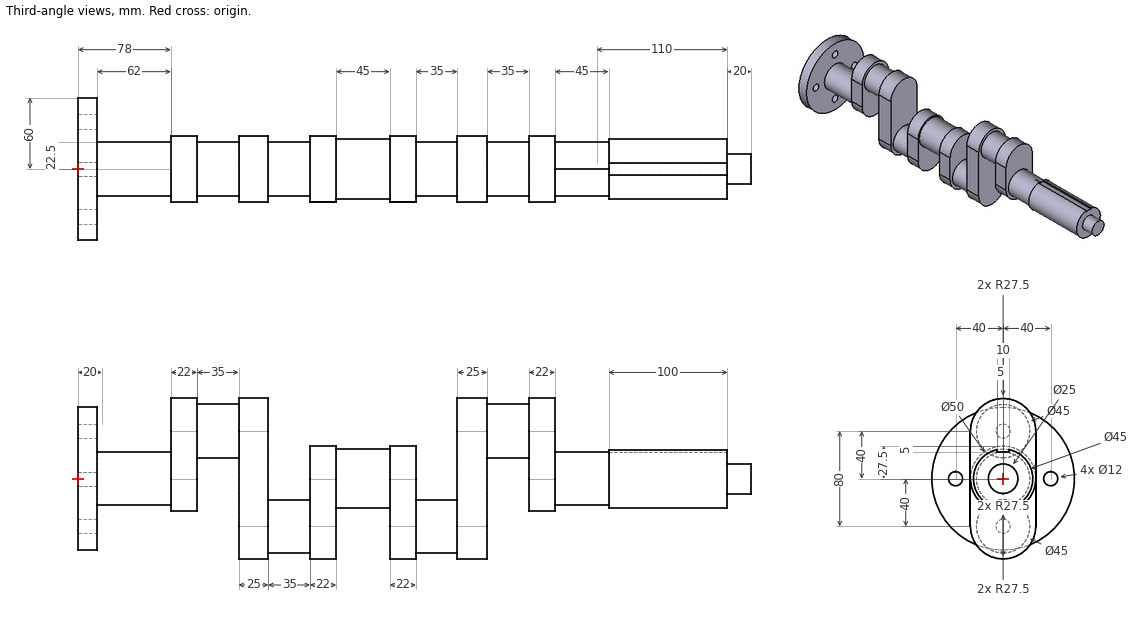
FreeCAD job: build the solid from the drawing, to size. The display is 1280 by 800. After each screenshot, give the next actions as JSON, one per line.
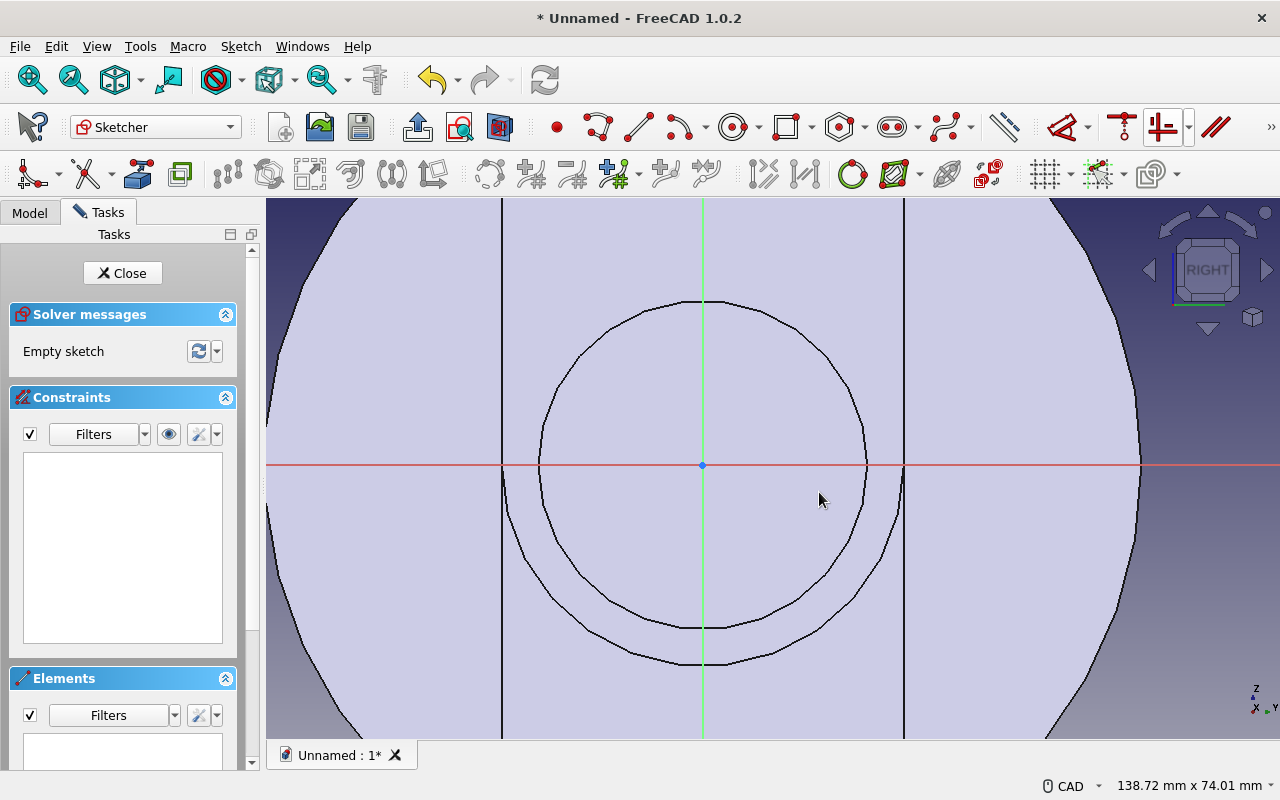
{"action": "left_click", "coordinate": [732, 128]}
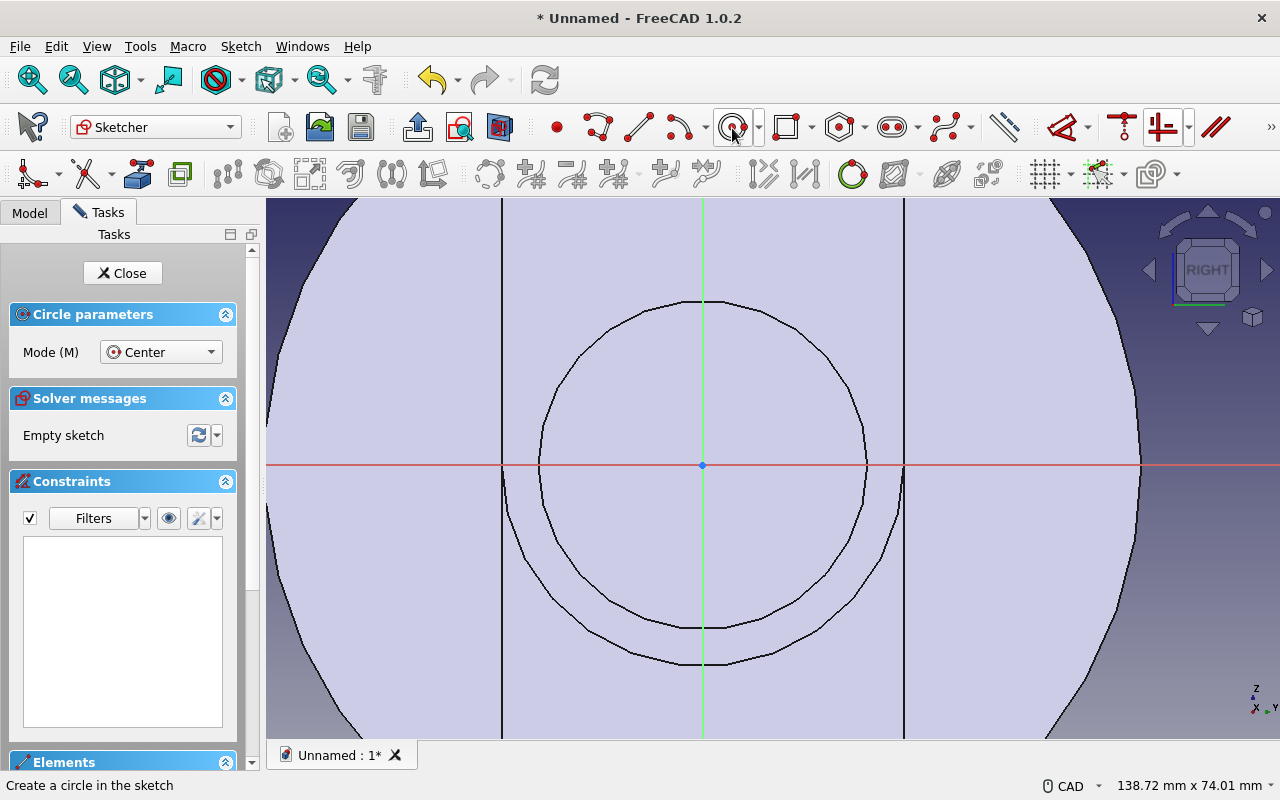
{"action": "left_click", "coordinate": [703, 465]}
{"action": "left_click", "coordinate": [832, 336]}
{"action": "key", "text": "Escape"}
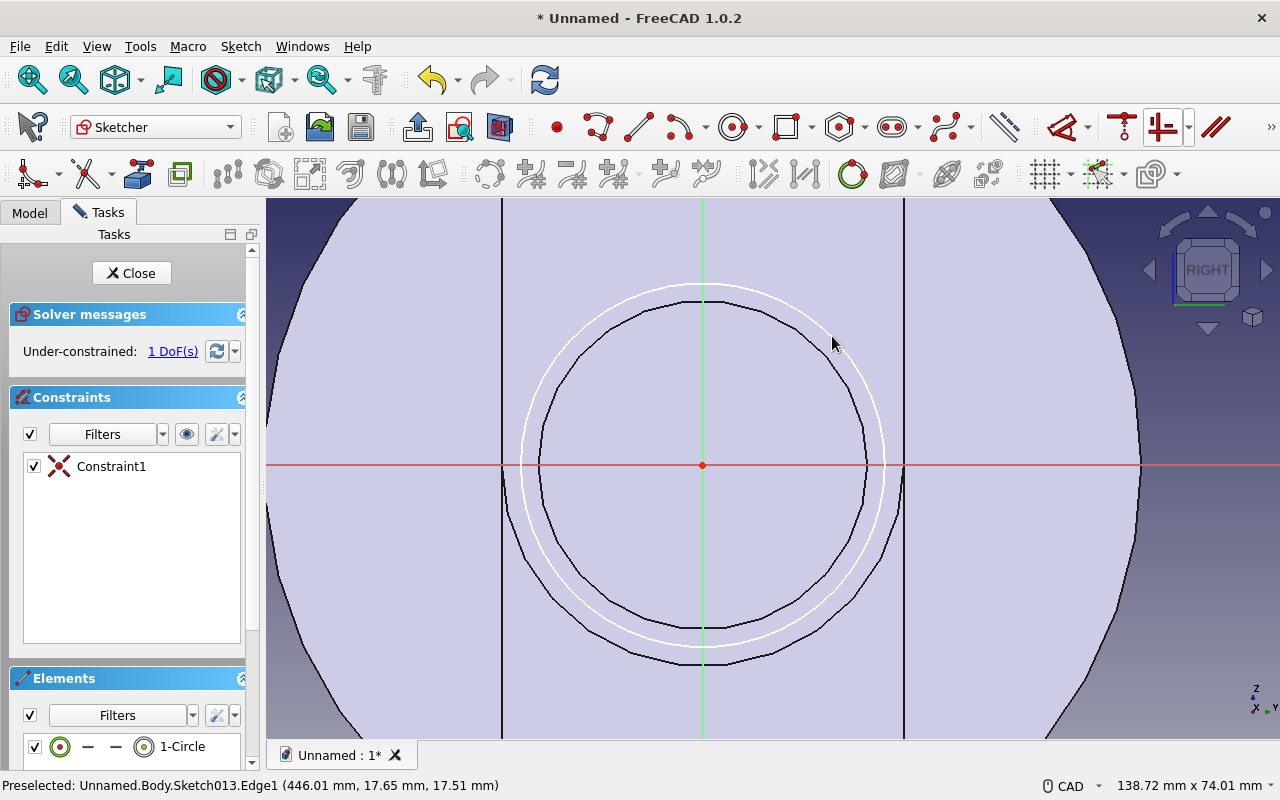
{"action": "key", "text": "d"}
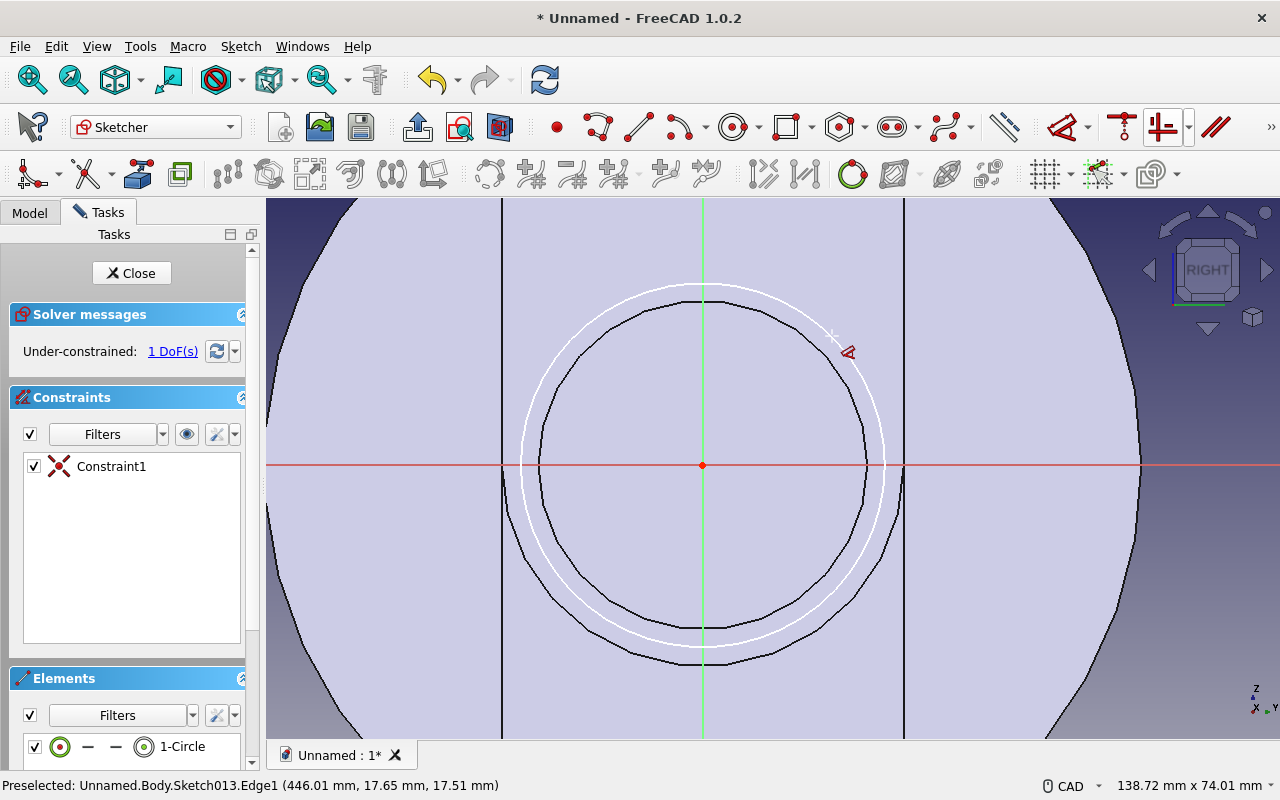
{"action": "left_click", "coordinate": [831, 336]}
{"action": "left_click", "coordinate": [854, 313]}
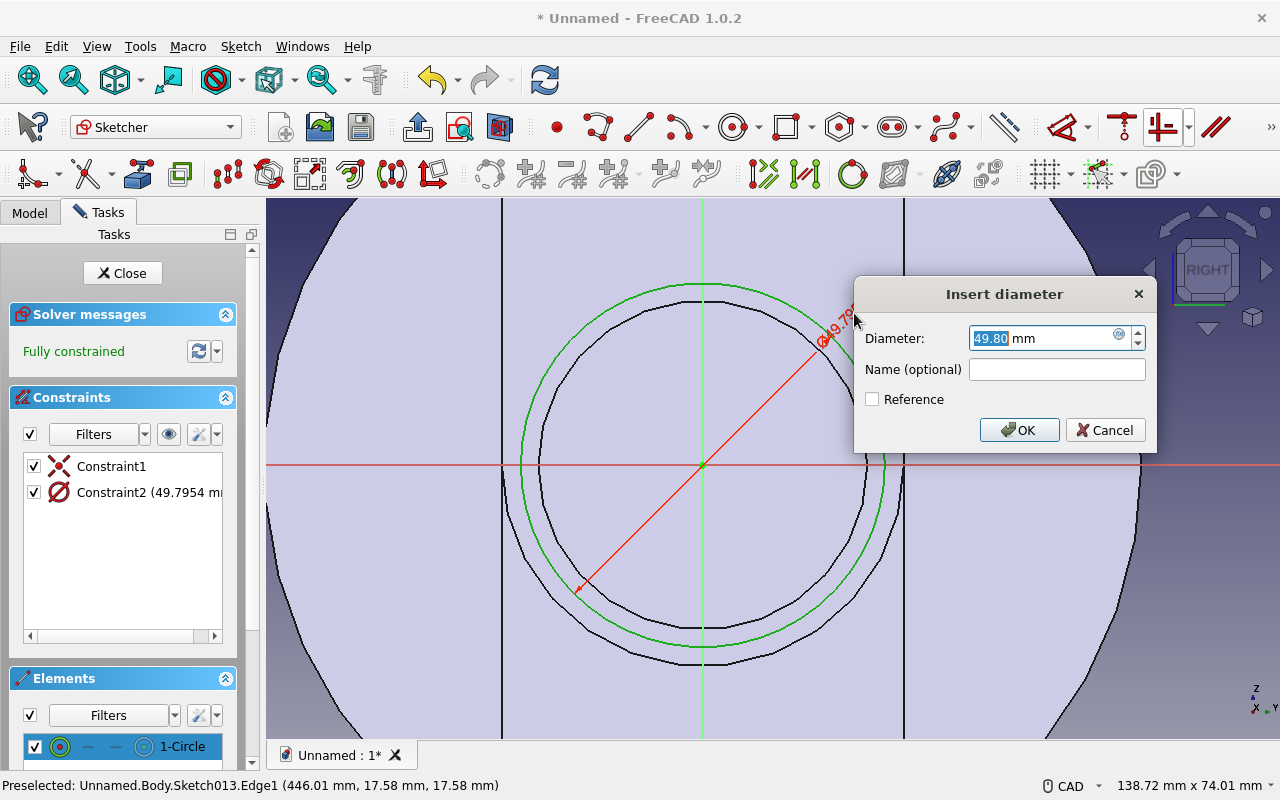
{"action": "type", "text": "50"}
{"action": "key", "text": "Return"}
{"action": "key", "text": "Escape"}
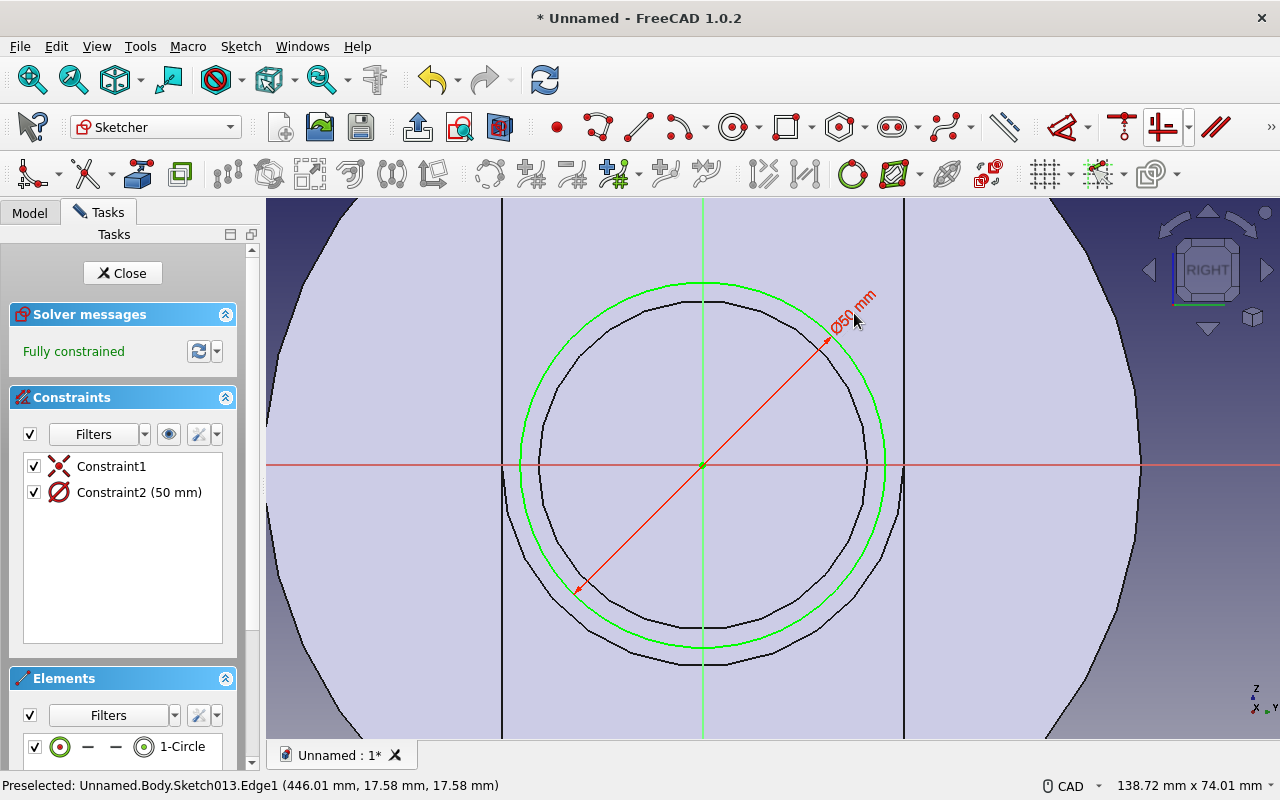
{"action": "left_click", "coordinate": [123, 273]}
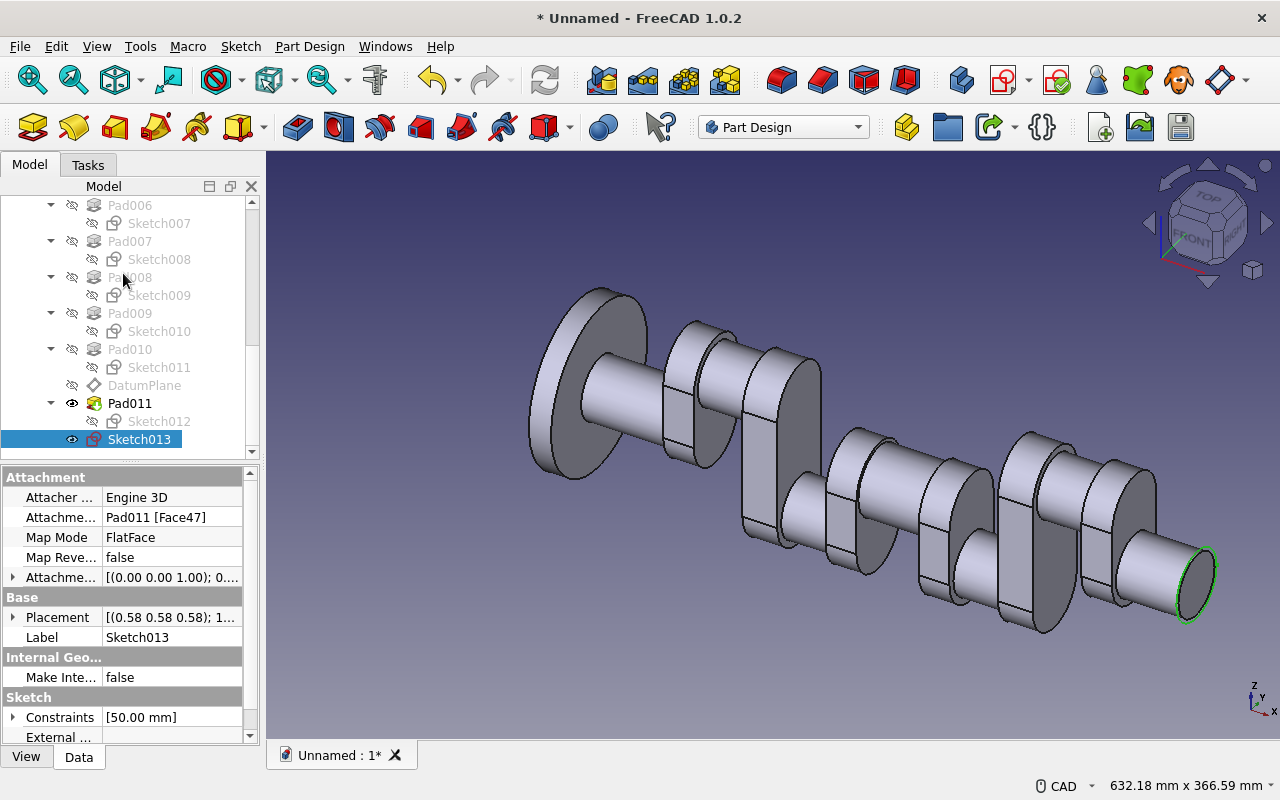
{"action": "left_click", "coordinate": [33, 128]}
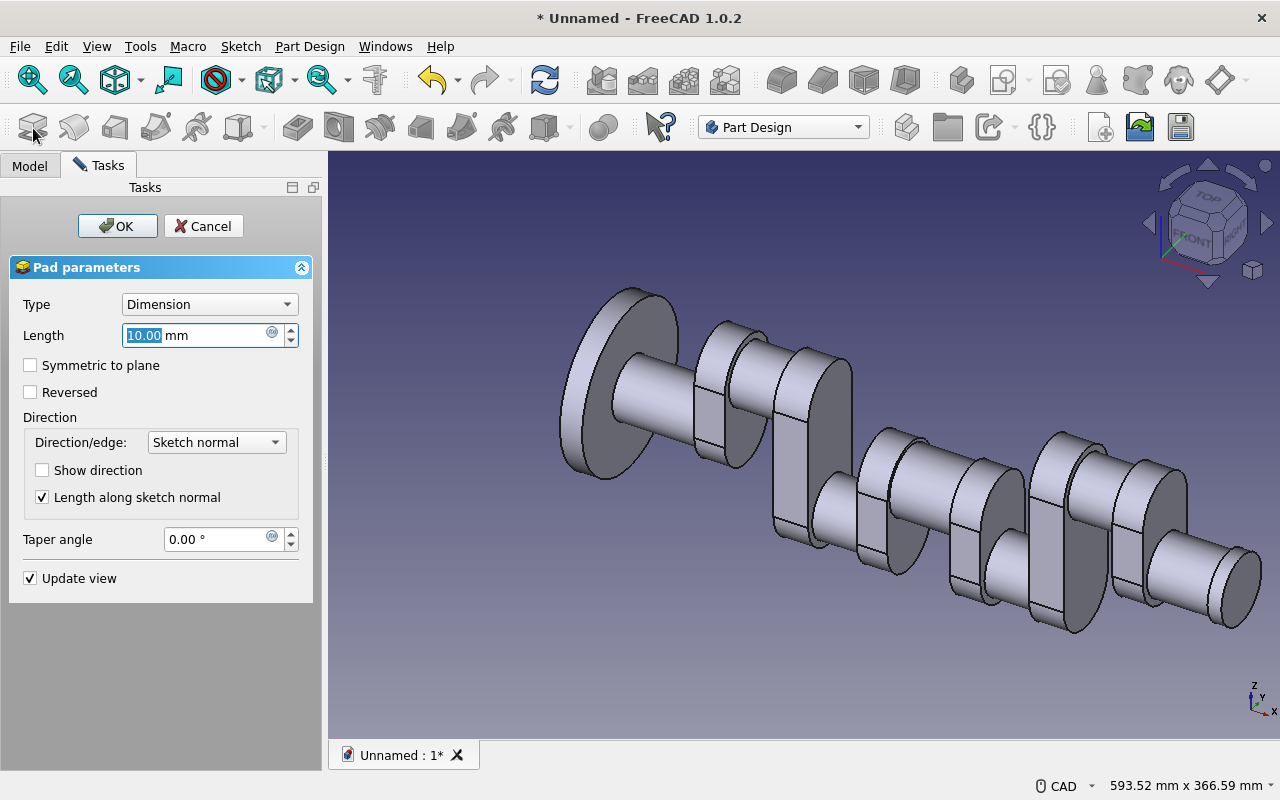
{"action": "type", "text": "100"}
{"action": "key", "text": "Tab"}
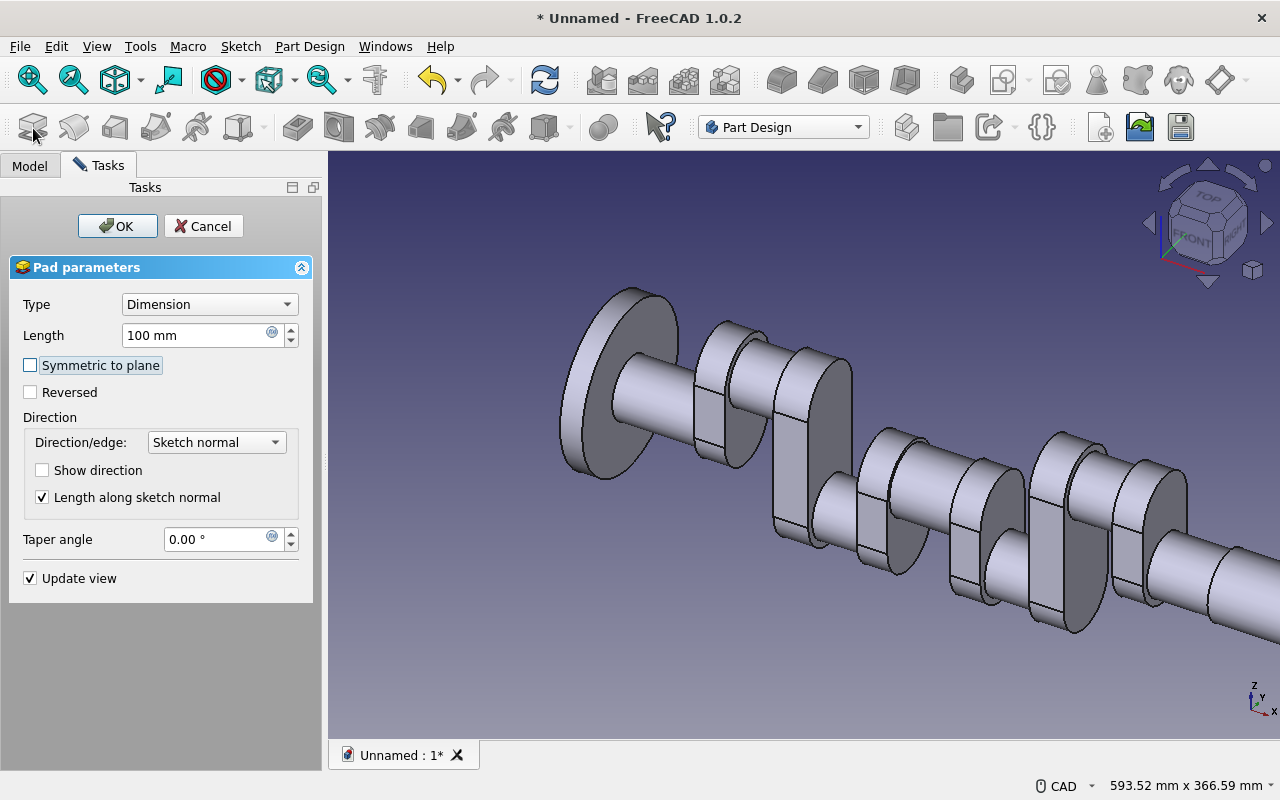
{"action": "left_click", "coordinate": [118, 226]}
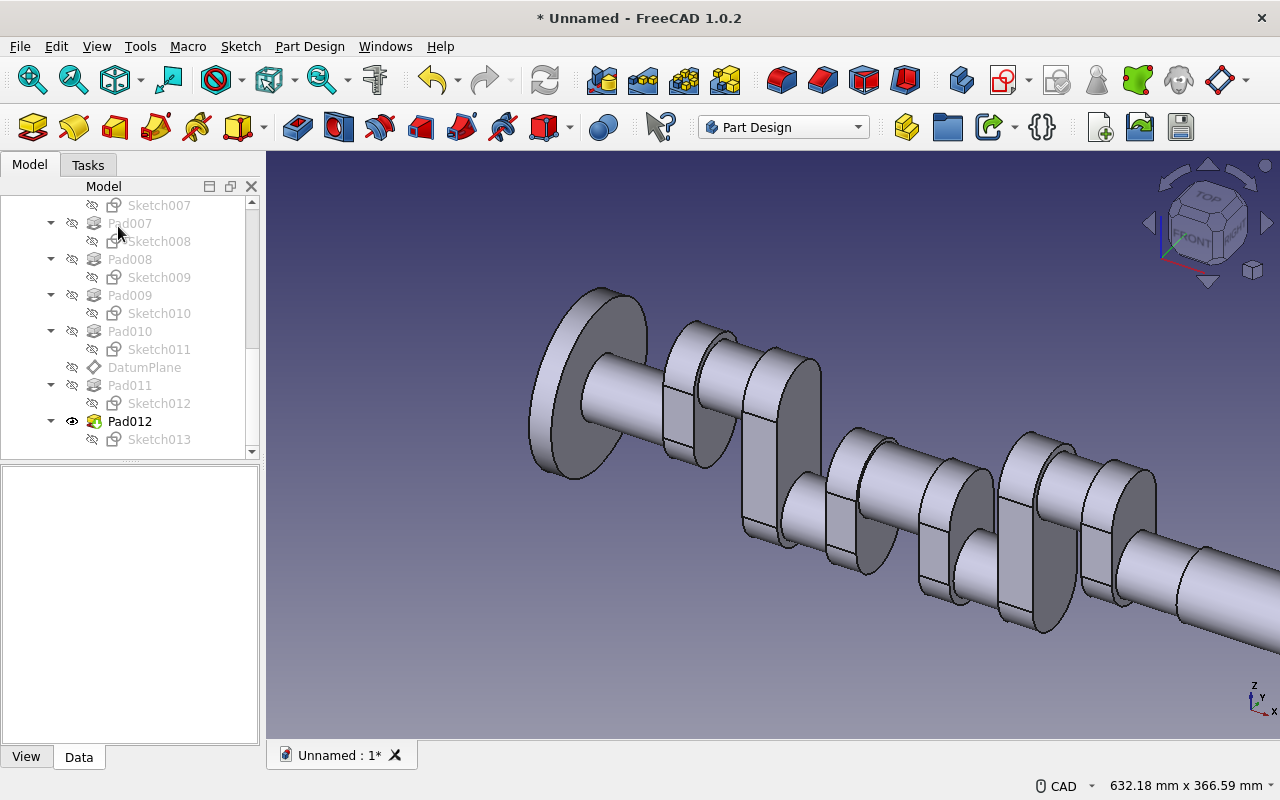
{"action": "left_click", "coordinate": [33, 80]}